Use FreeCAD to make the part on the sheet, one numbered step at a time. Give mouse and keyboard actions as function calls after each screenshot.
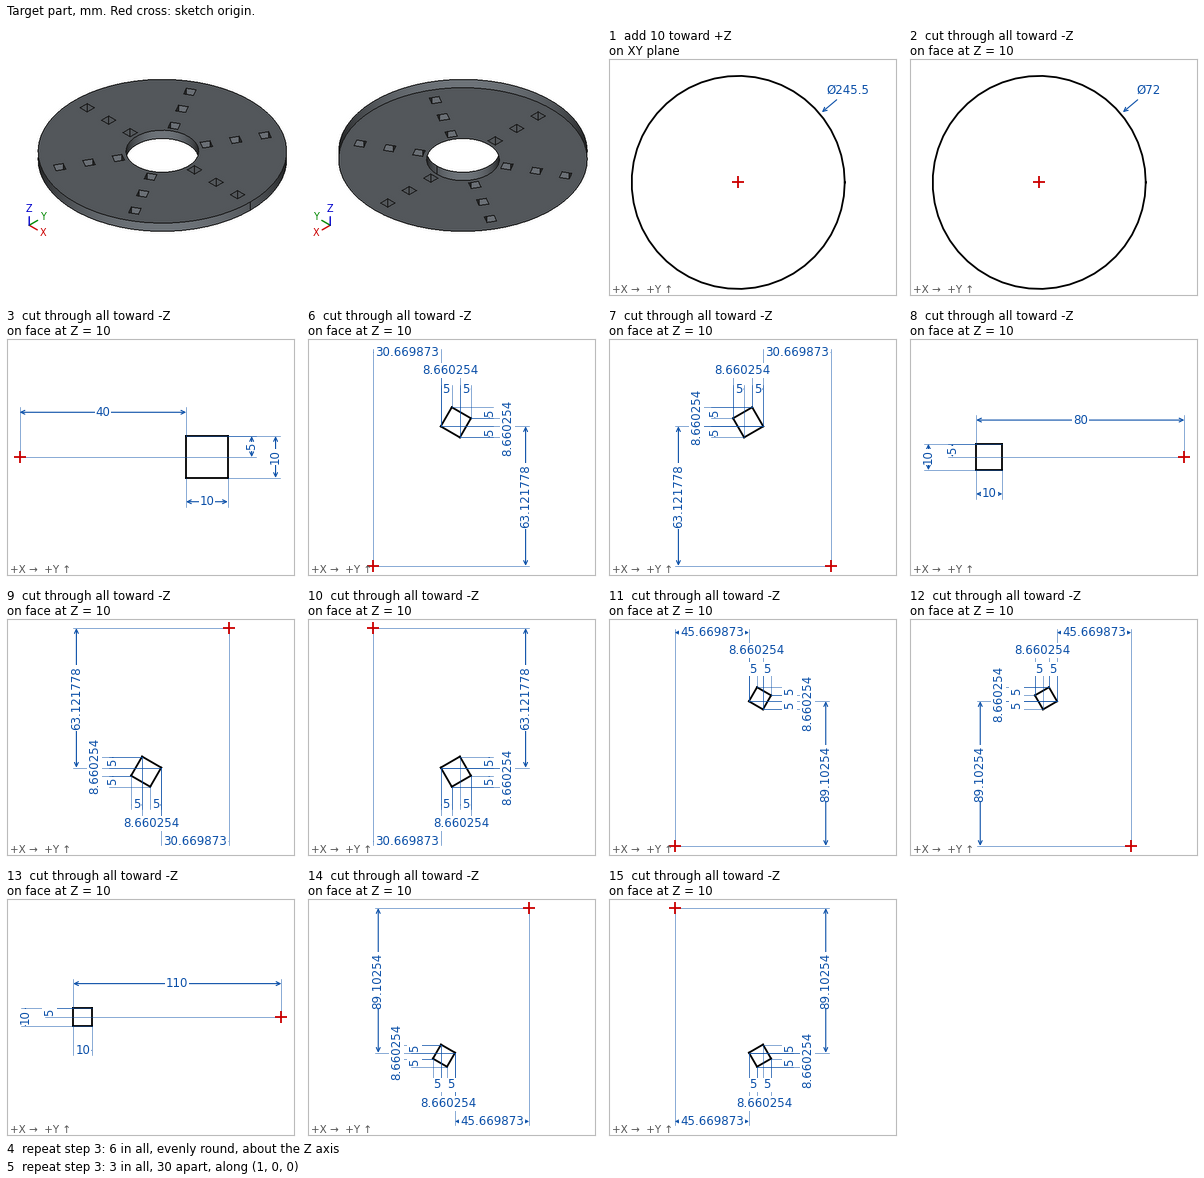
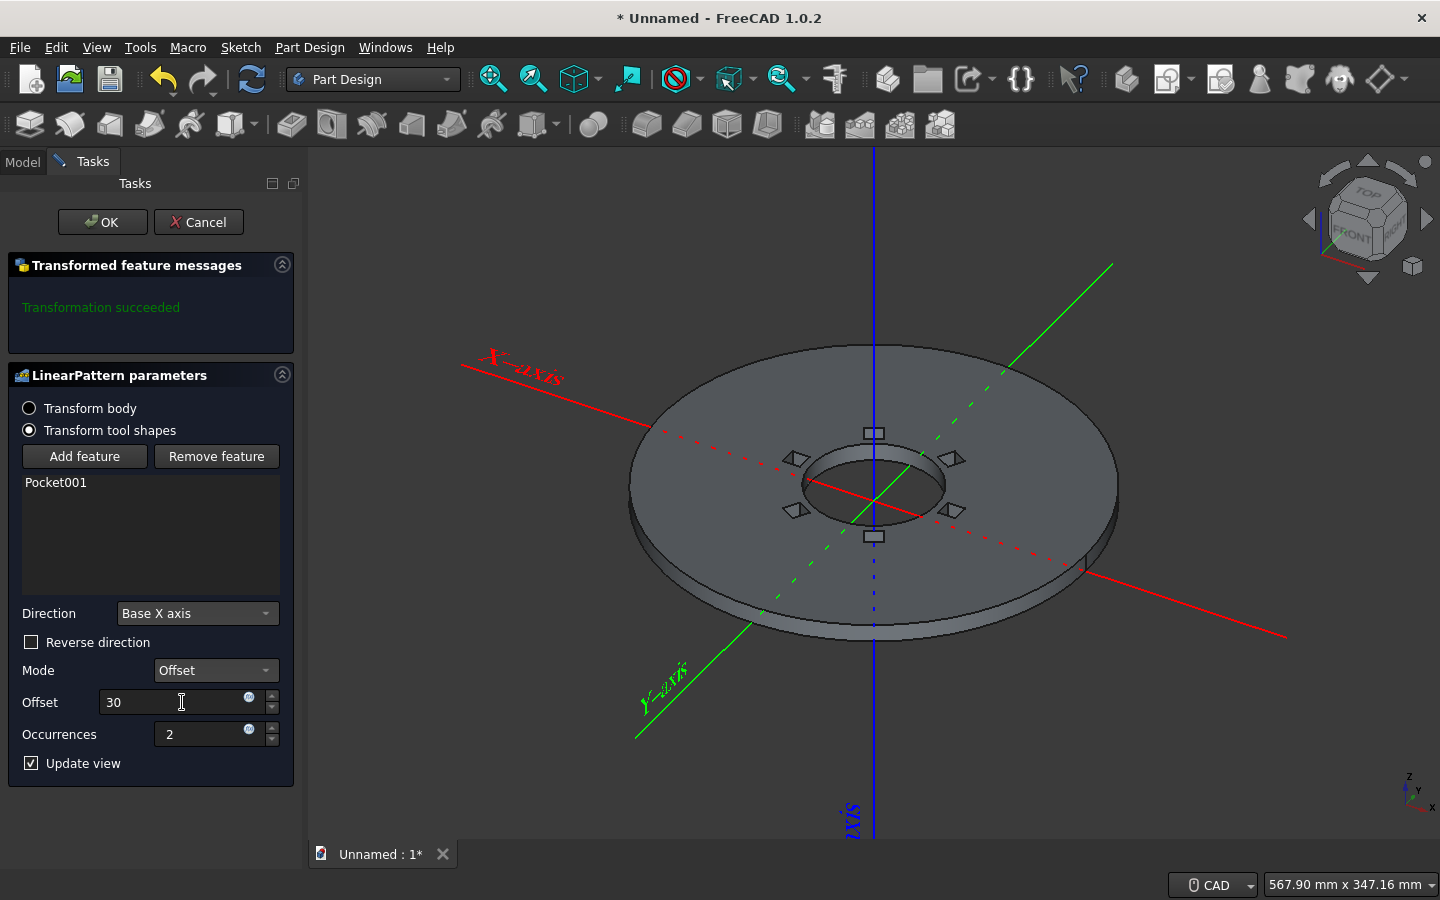
triple_click(209, 734)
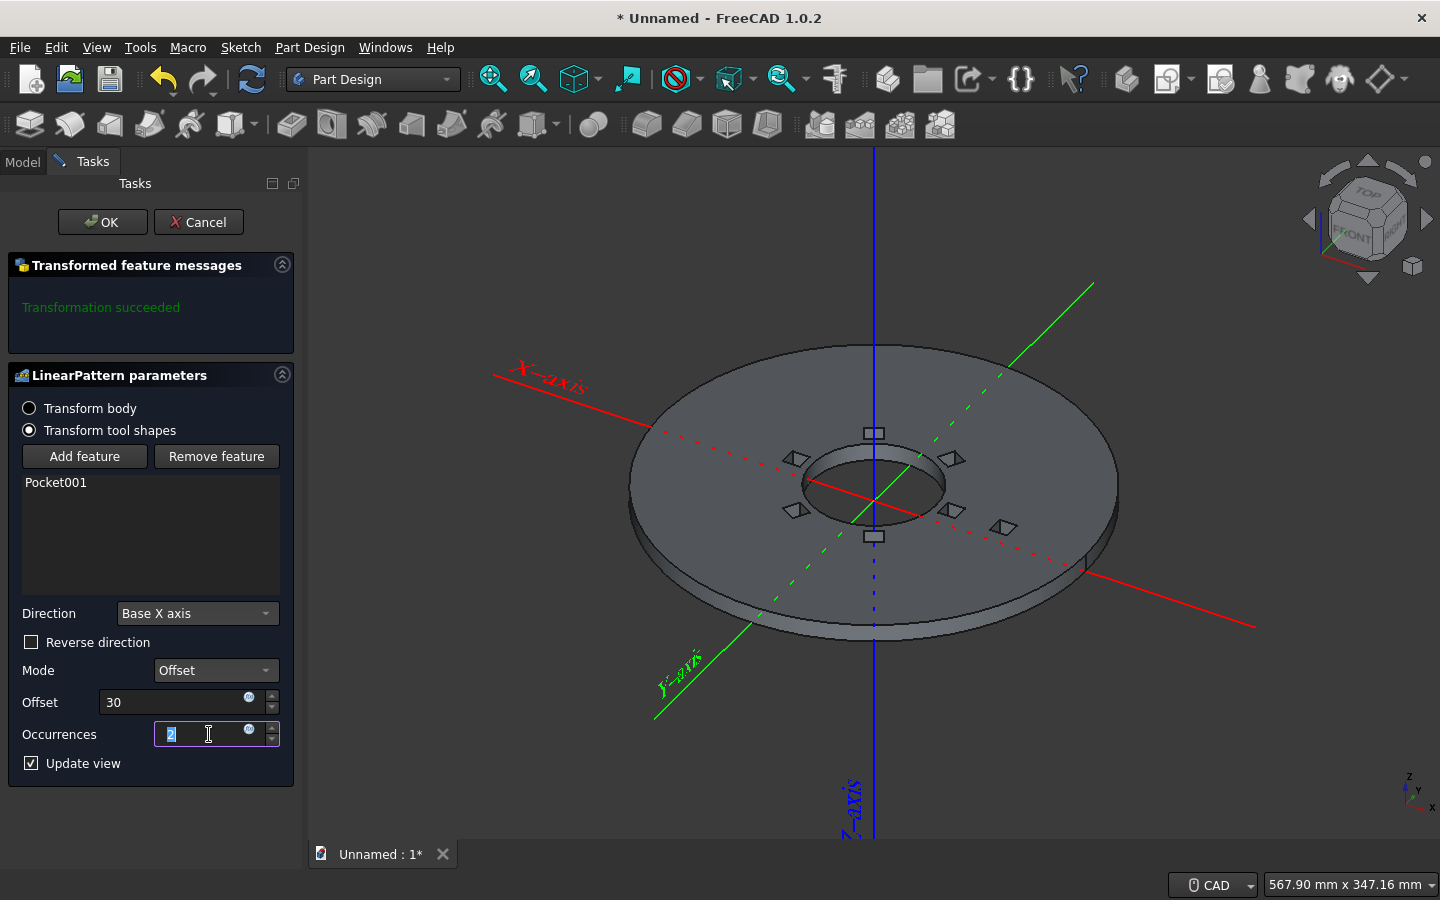
text(3)
key(Tab)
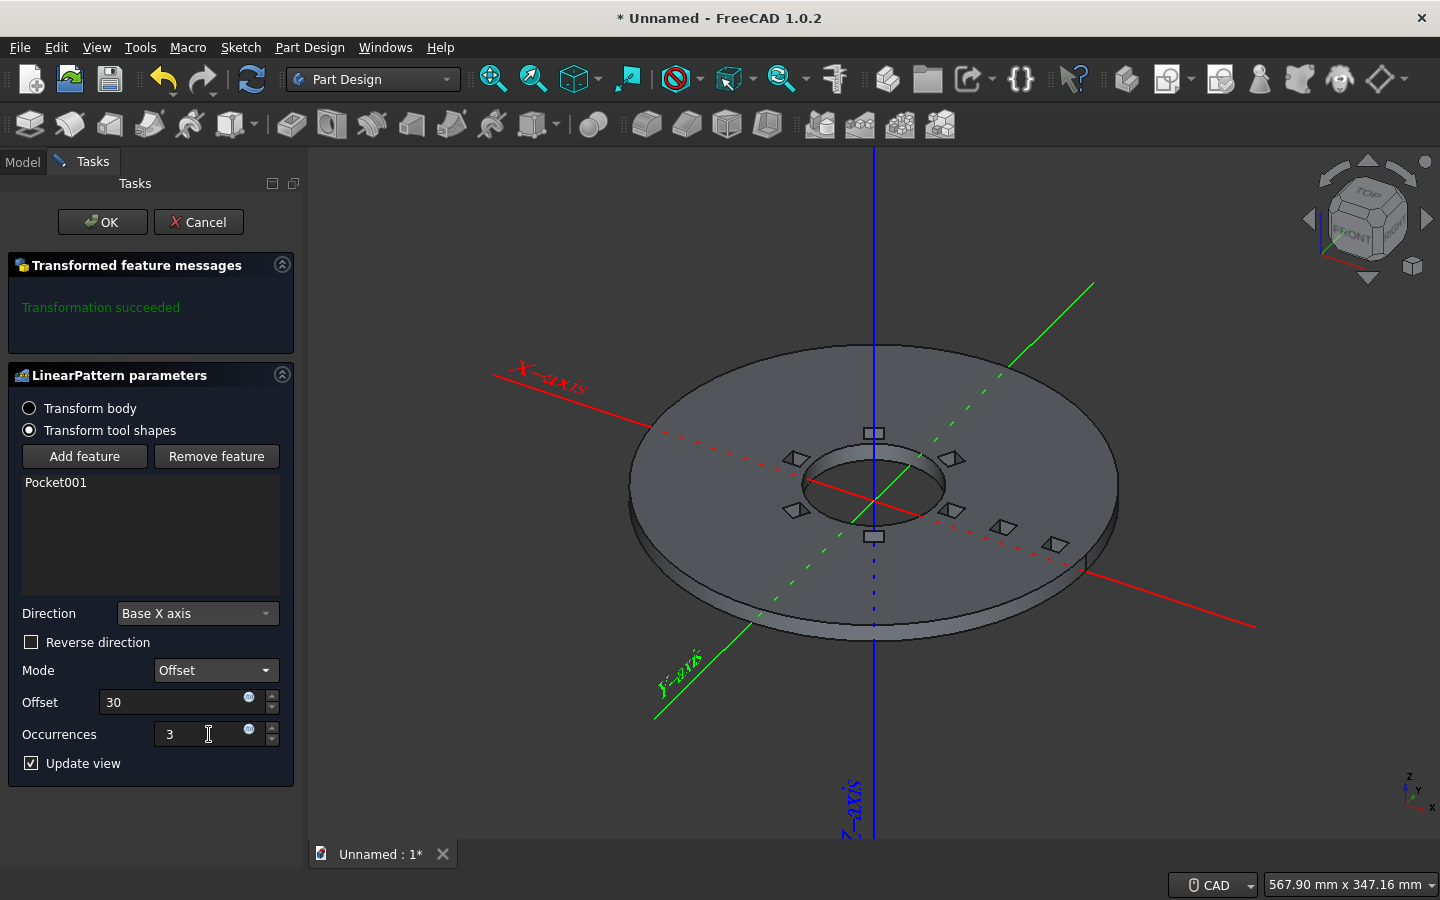
click(103, 222)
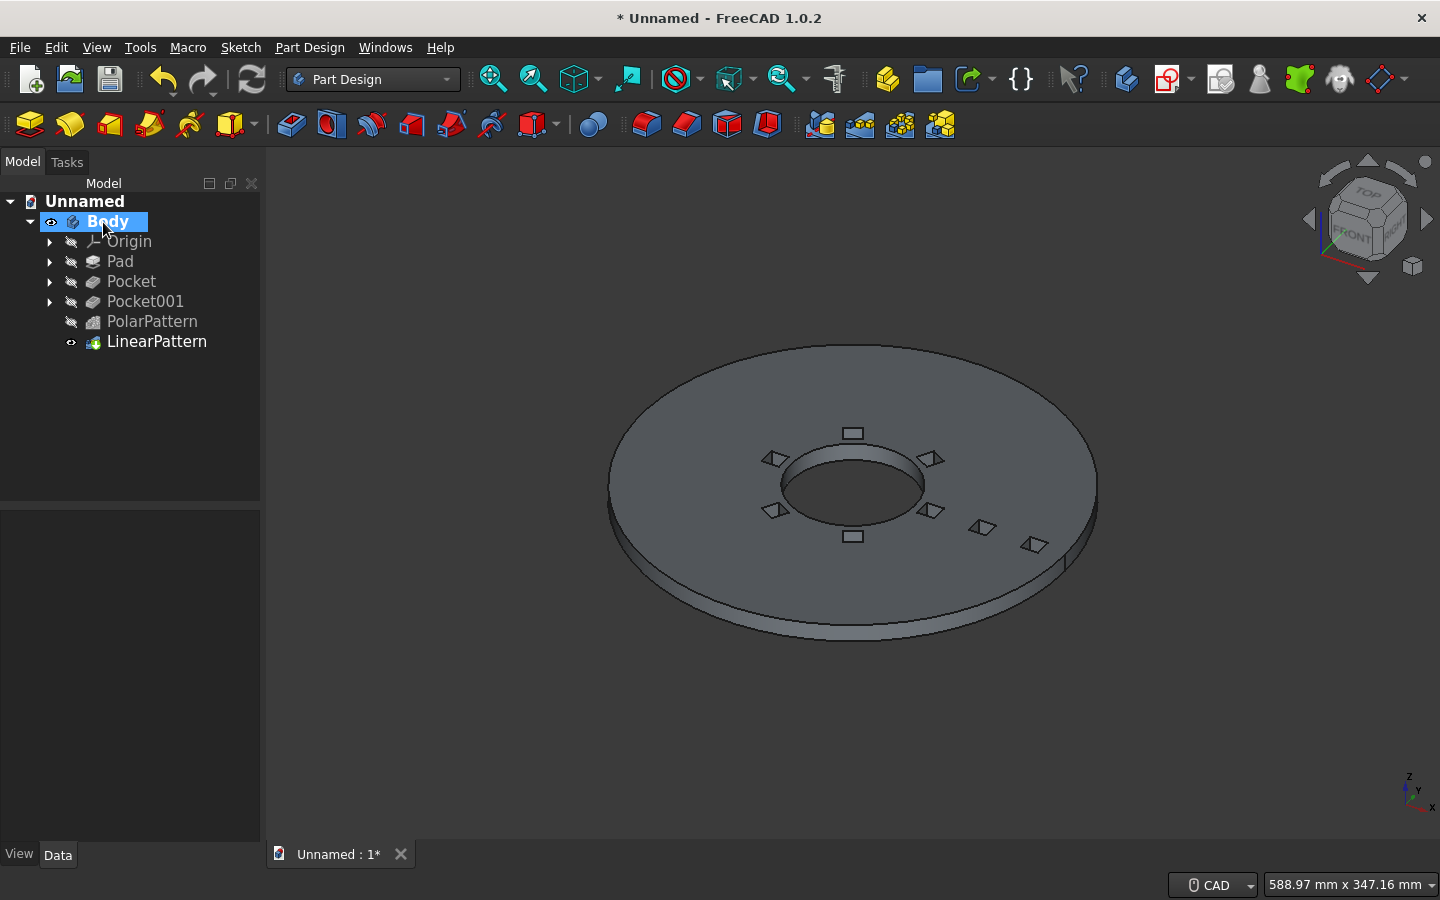
click(767, 409)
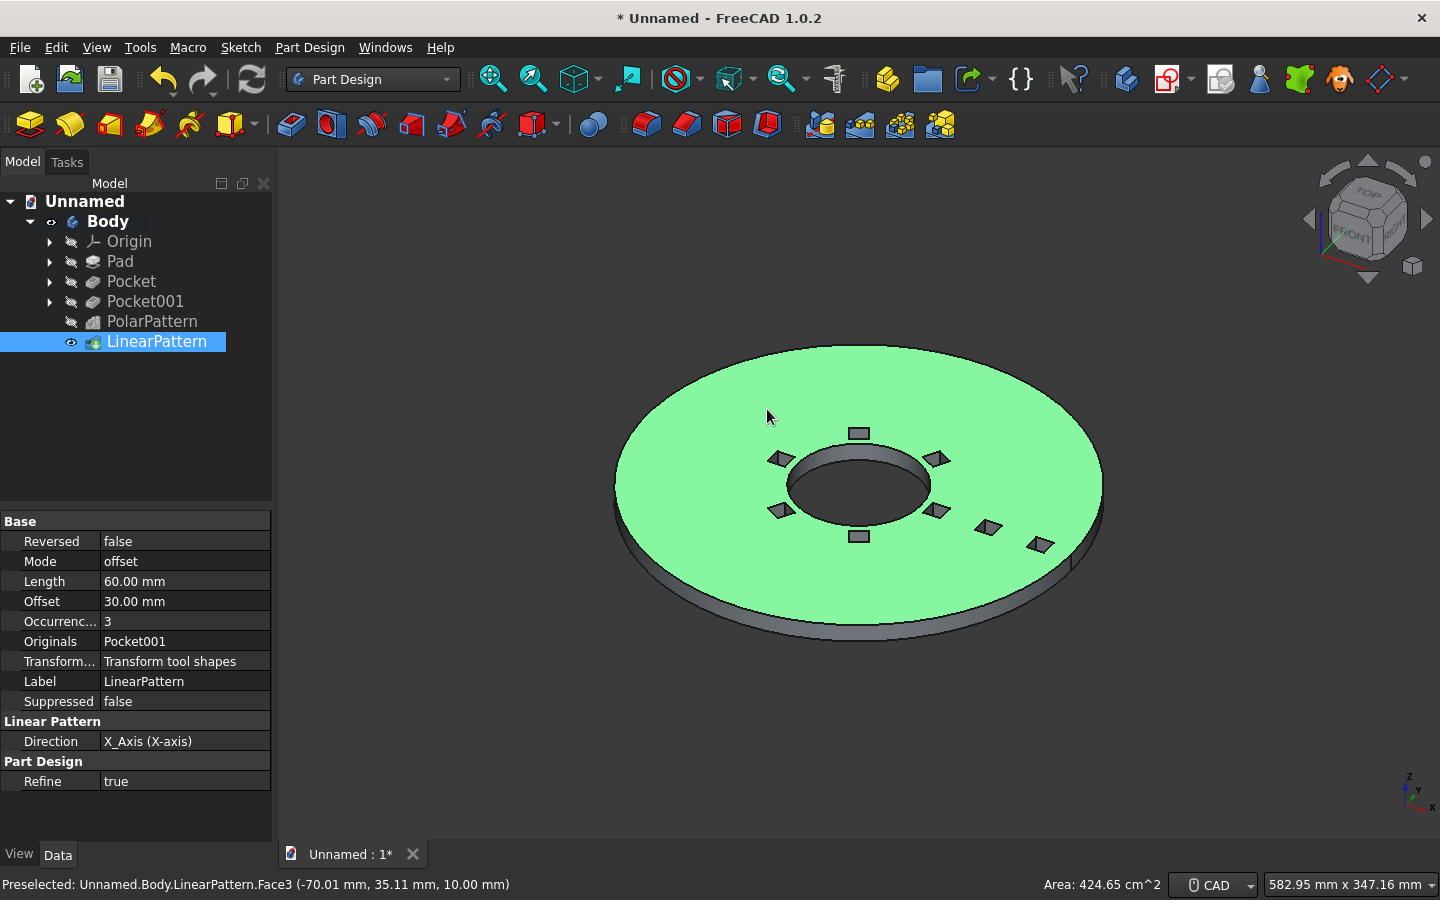
click(1168, 80)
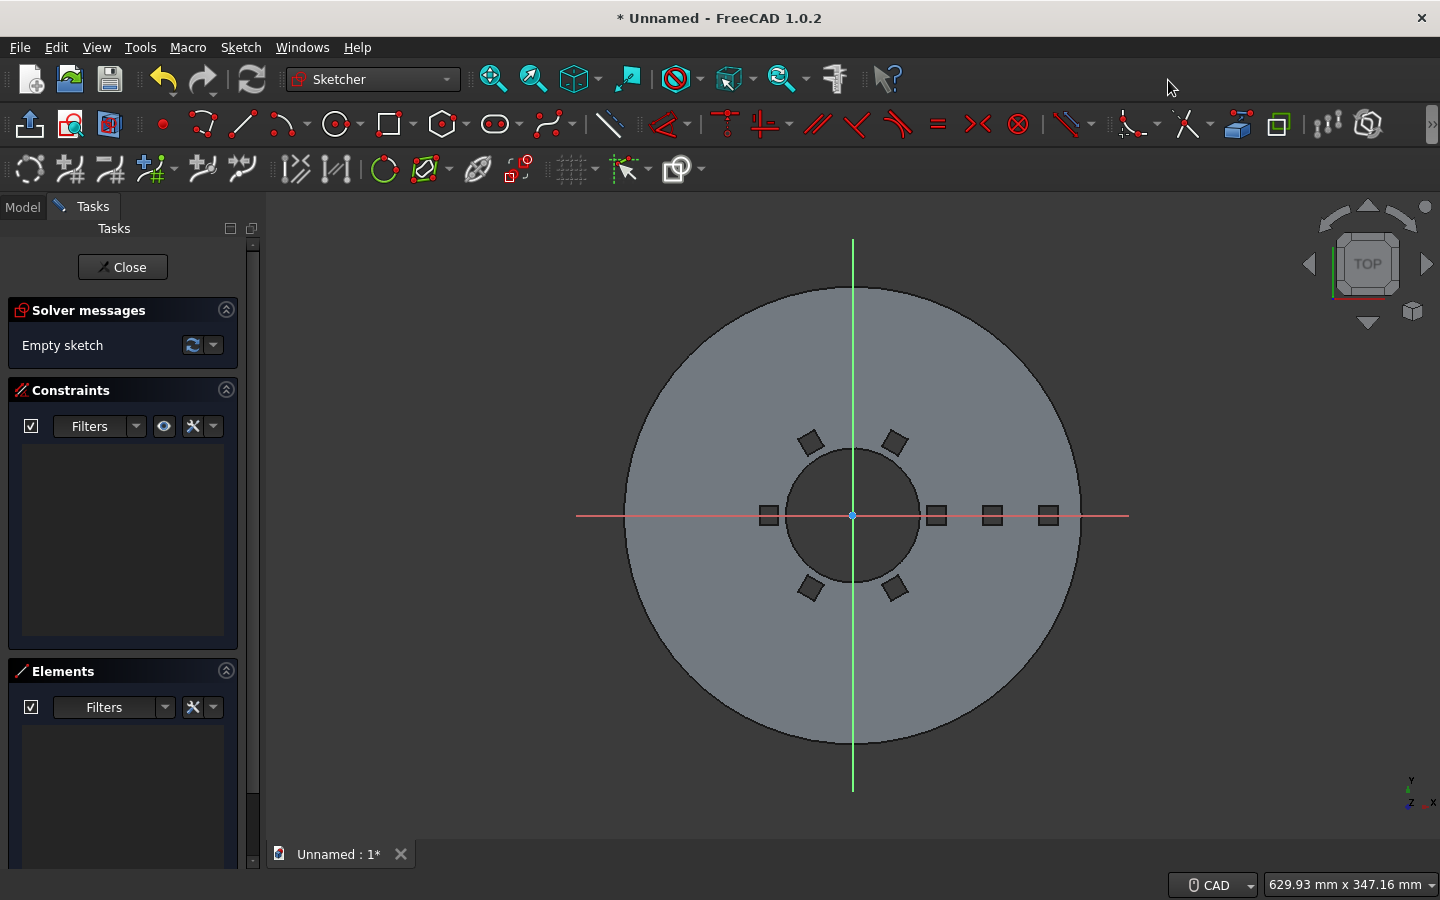
scroll(932, 387, up, 14)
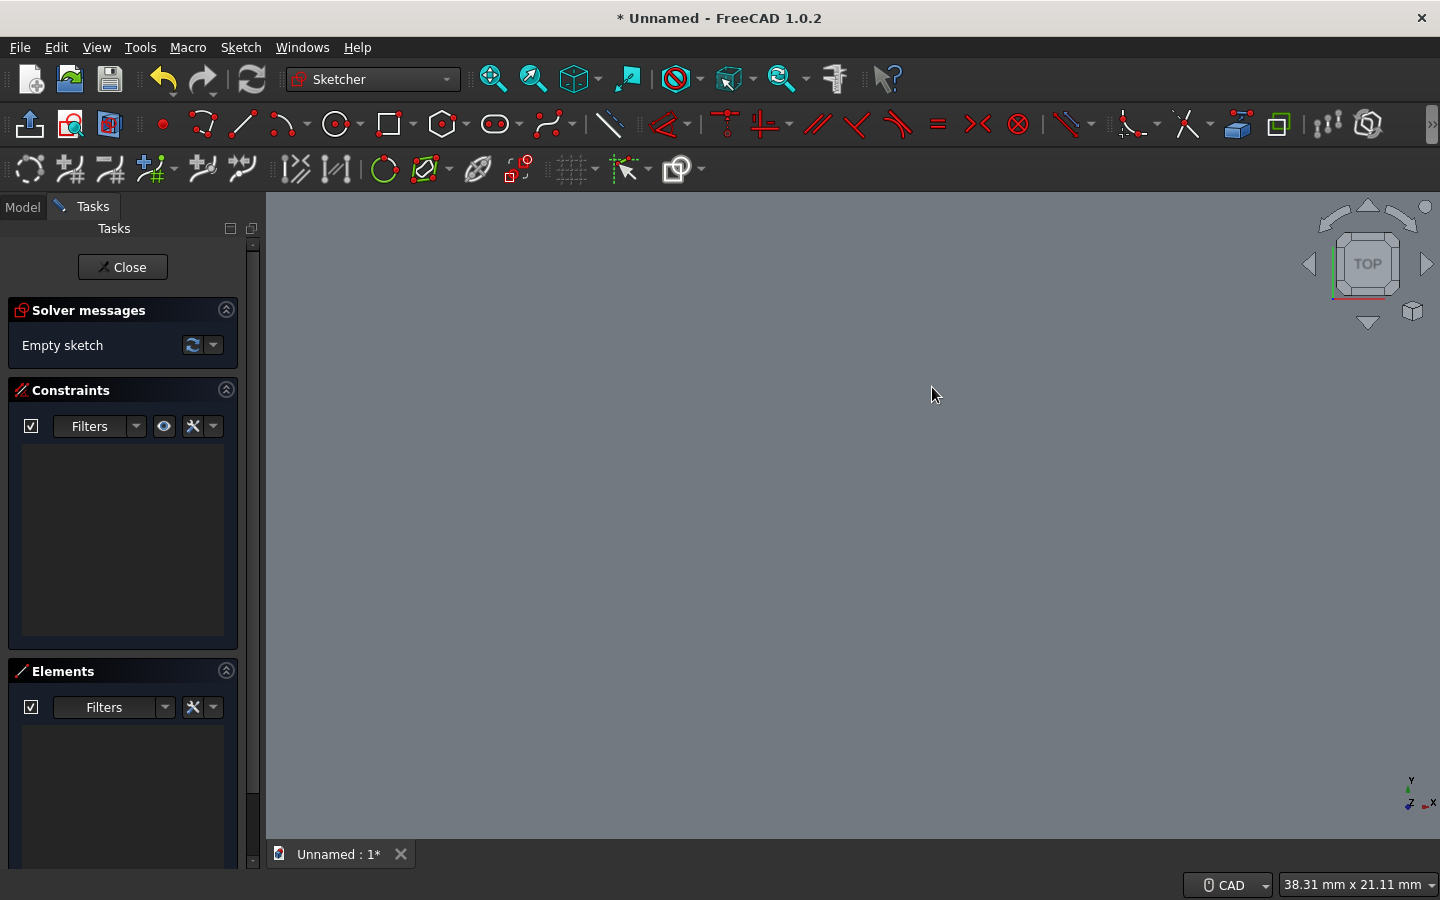
key(g)
key(m)